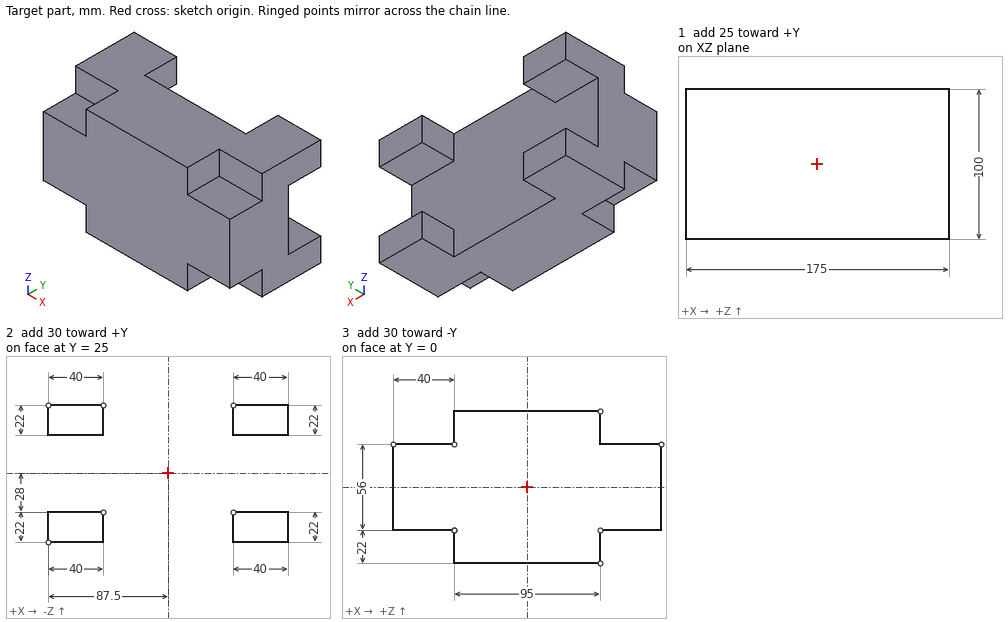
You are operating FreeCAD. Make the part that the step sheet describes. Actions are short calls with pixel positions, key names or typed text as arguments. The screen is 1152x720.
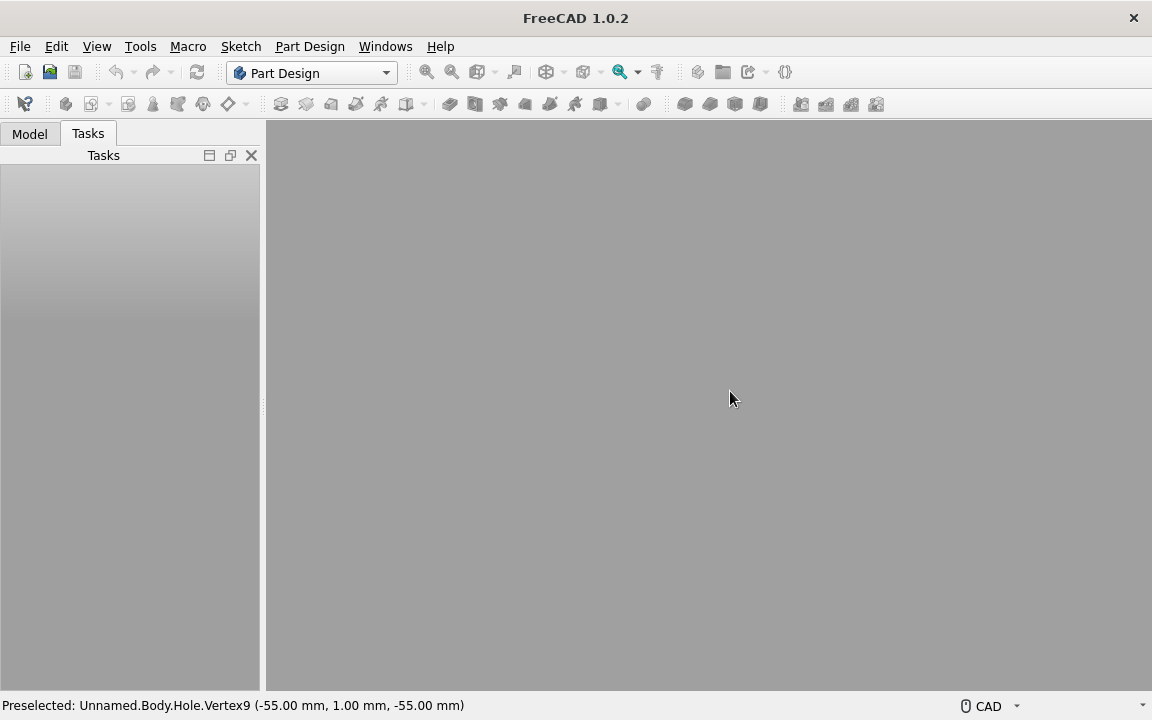
click(25, 72)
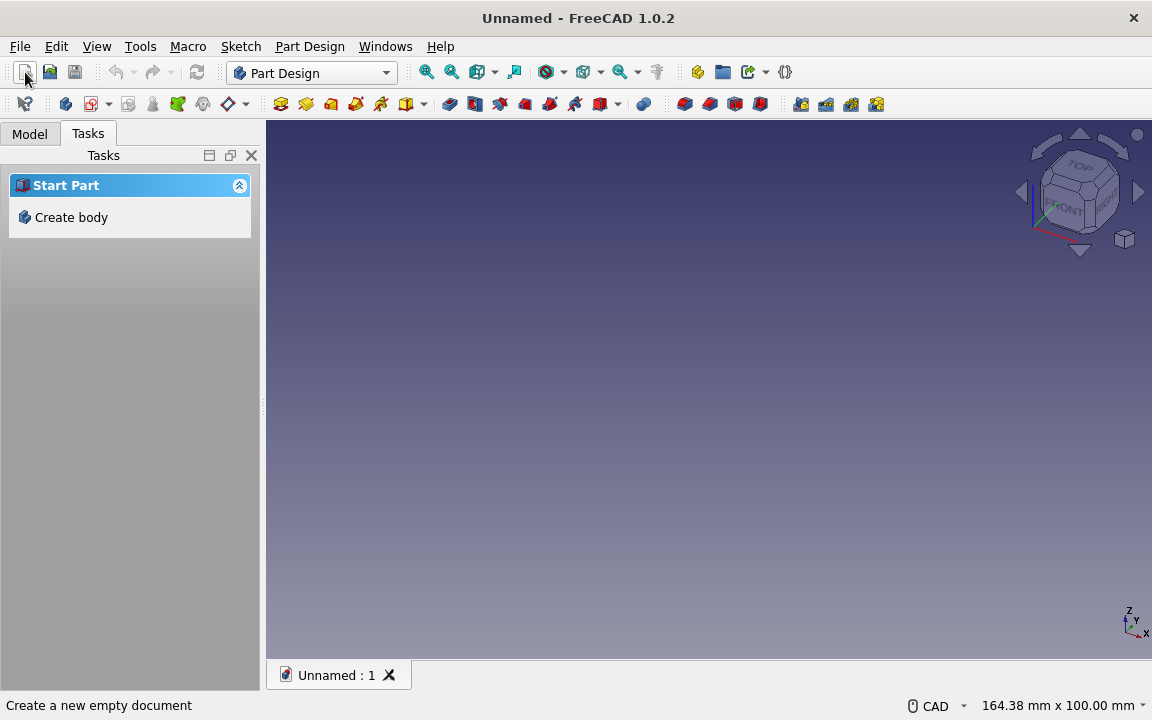
click(90, 104)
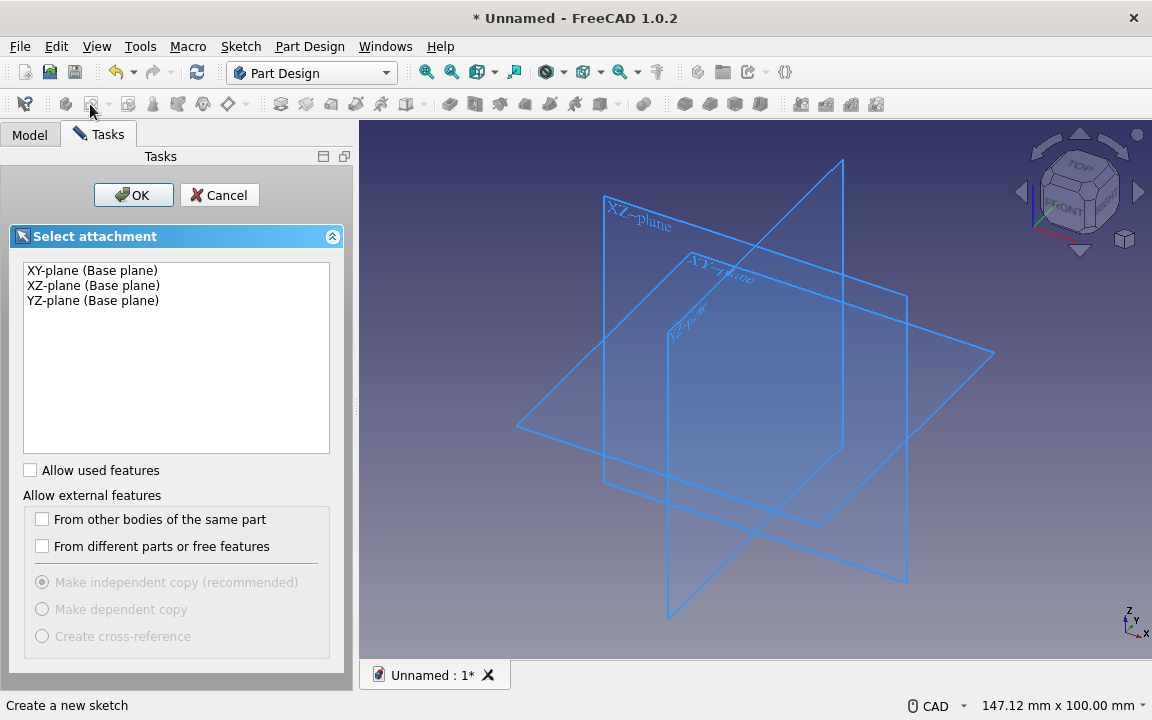
click(84, 286)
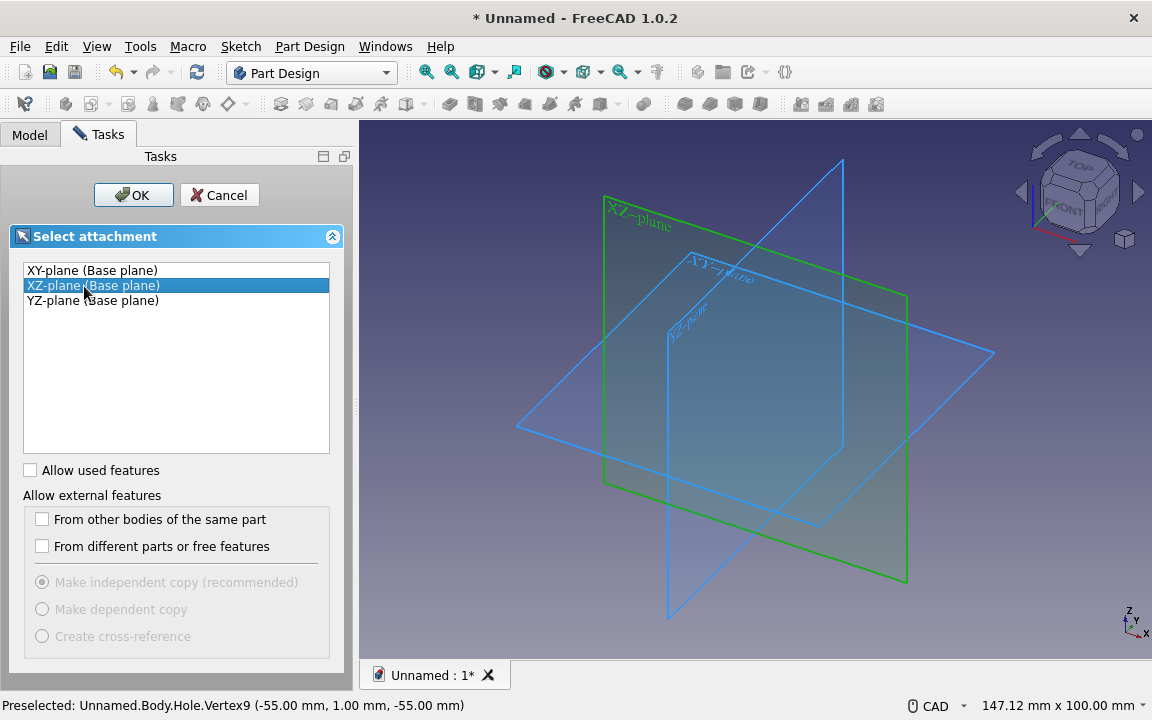
click(134, 195)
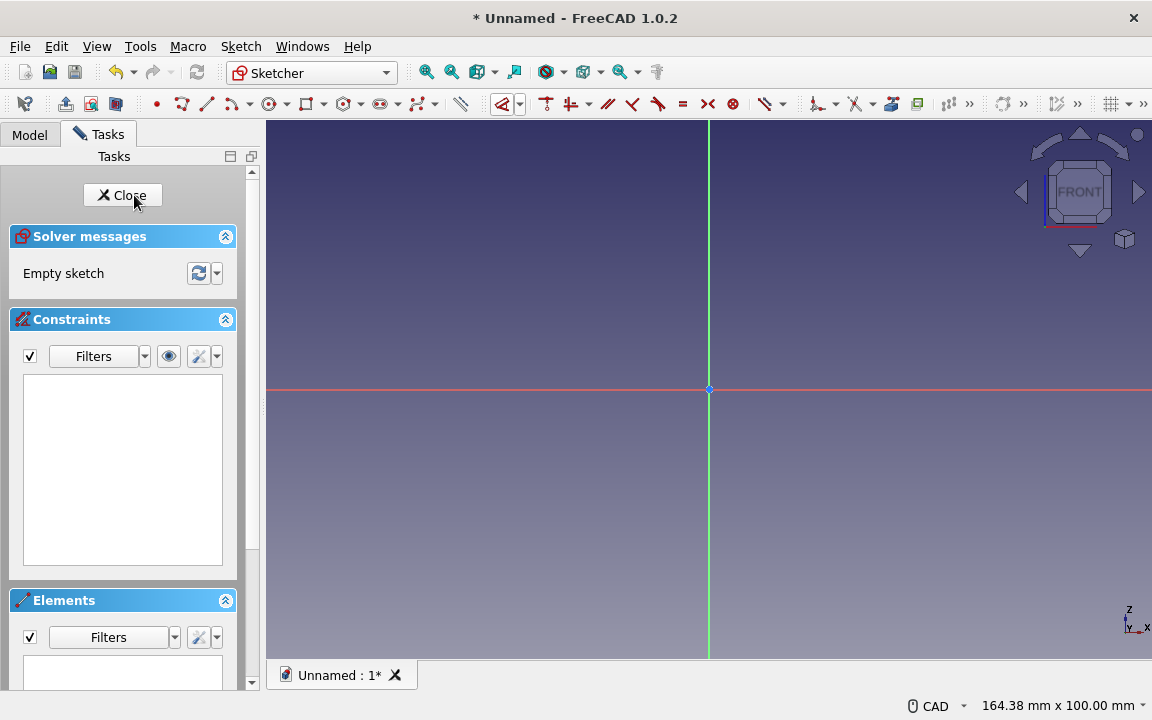
scroll(557, 390, down, 3)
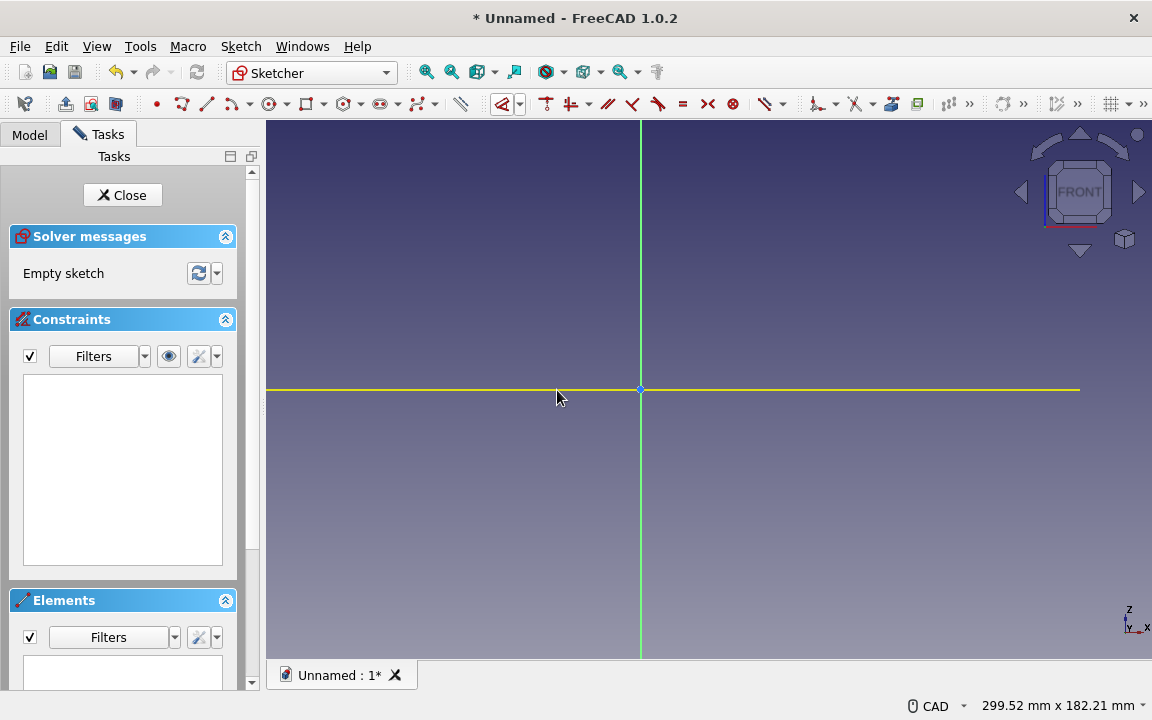
key(g)
key(v)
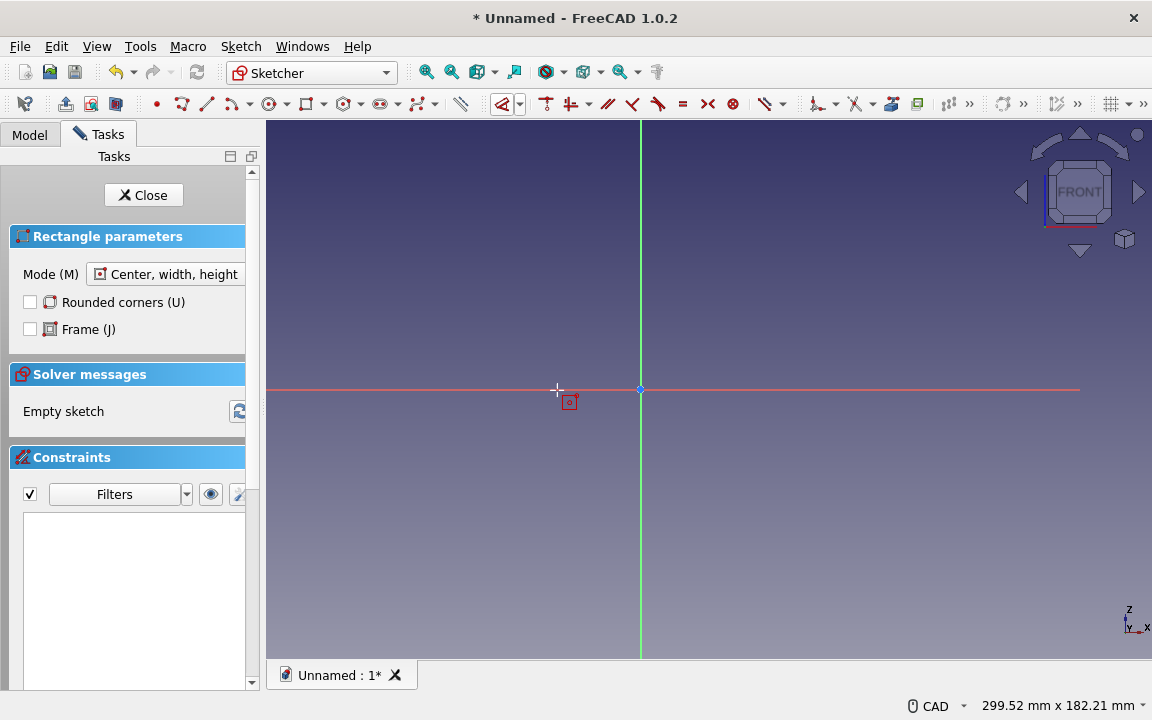
click(641, 390)
move(899, 242)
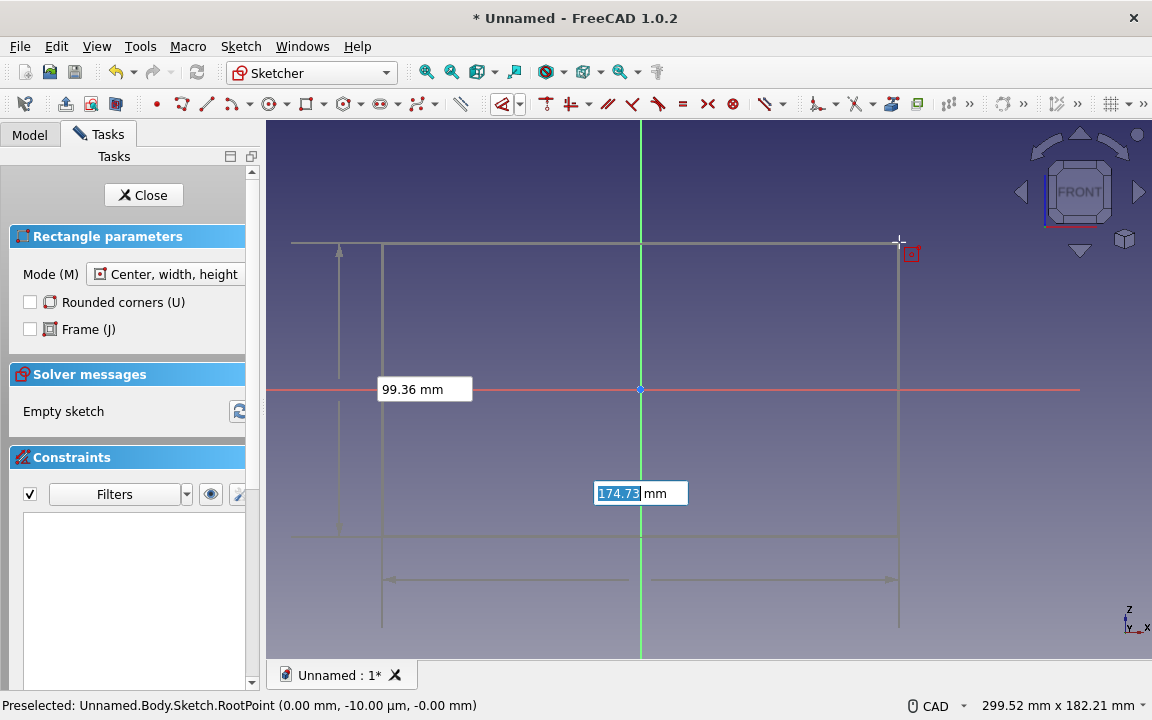
text(175)
key(Tab)
text(100)
key(Return)
key(Escape)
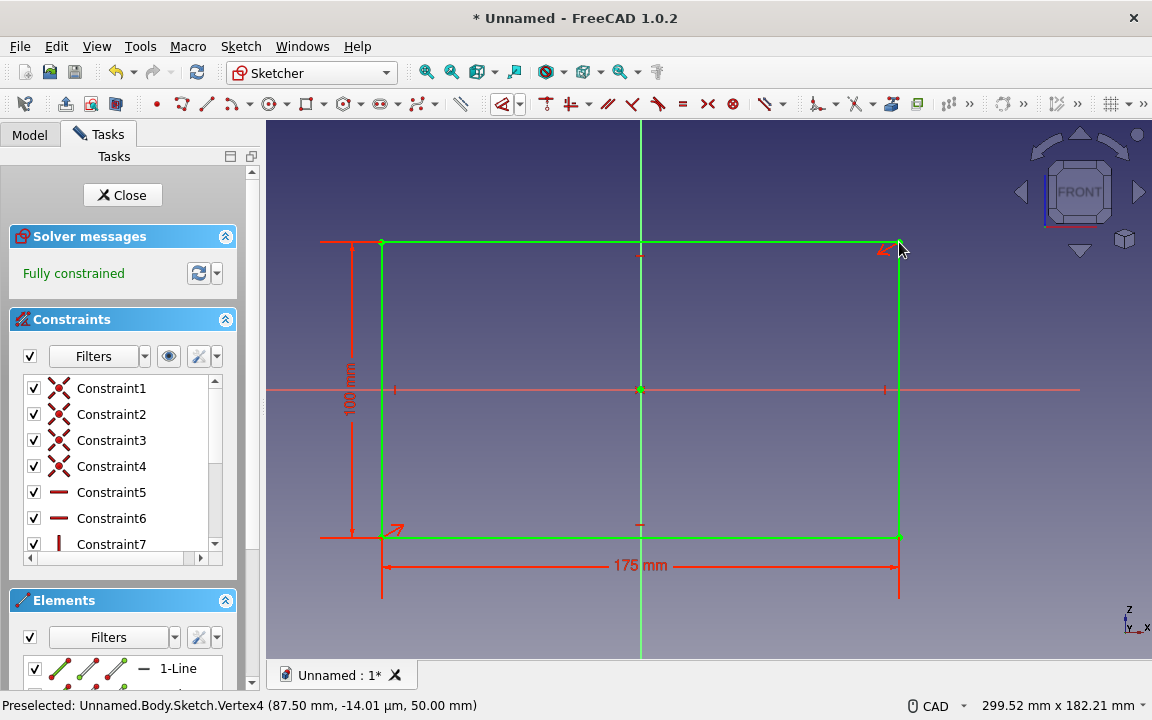
click(123, 195)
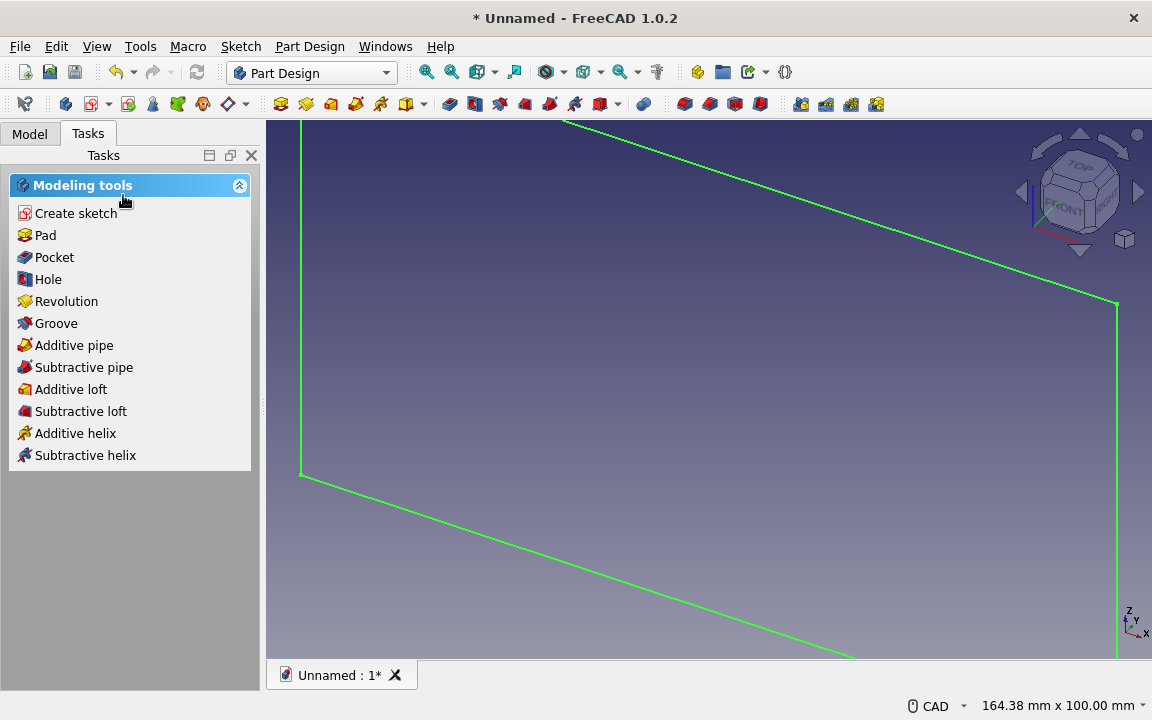
click(281, 104)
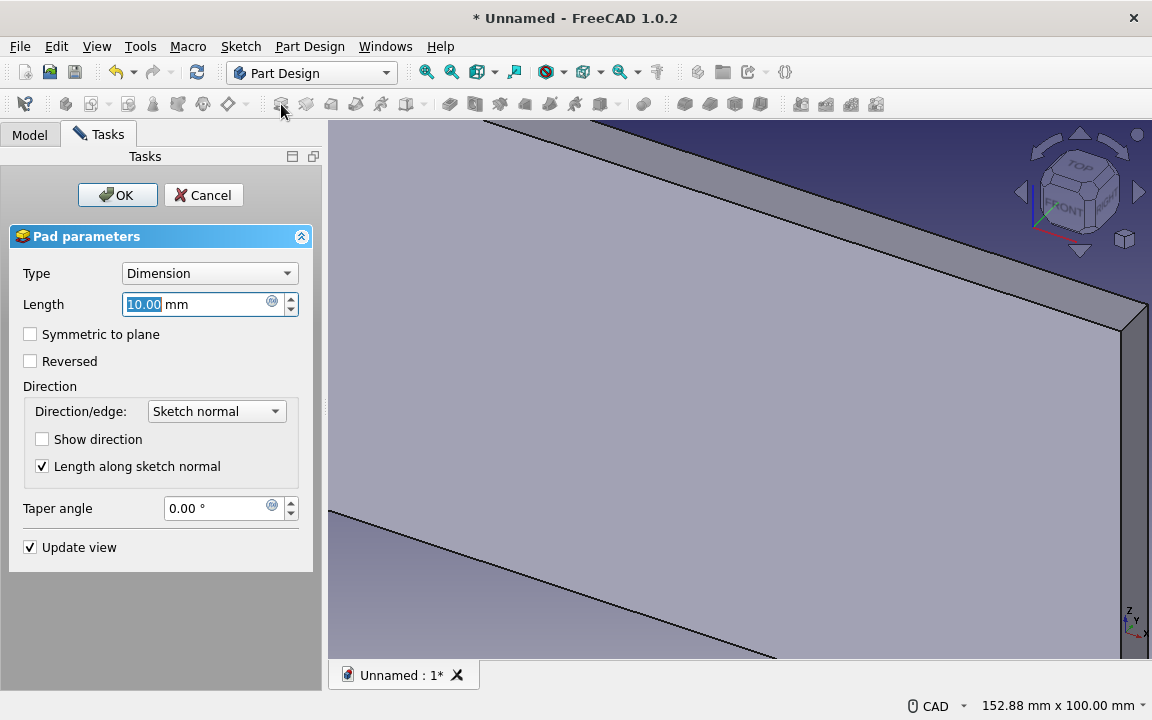
text(25)
key(Tab)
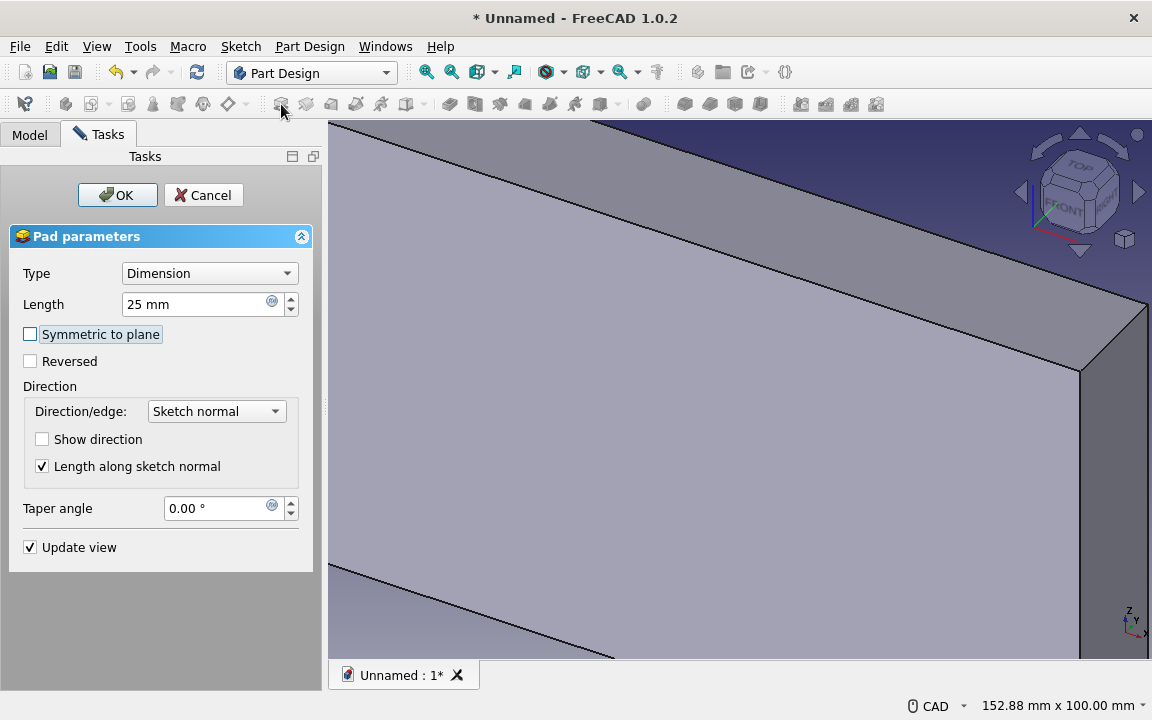
click(31, 361)